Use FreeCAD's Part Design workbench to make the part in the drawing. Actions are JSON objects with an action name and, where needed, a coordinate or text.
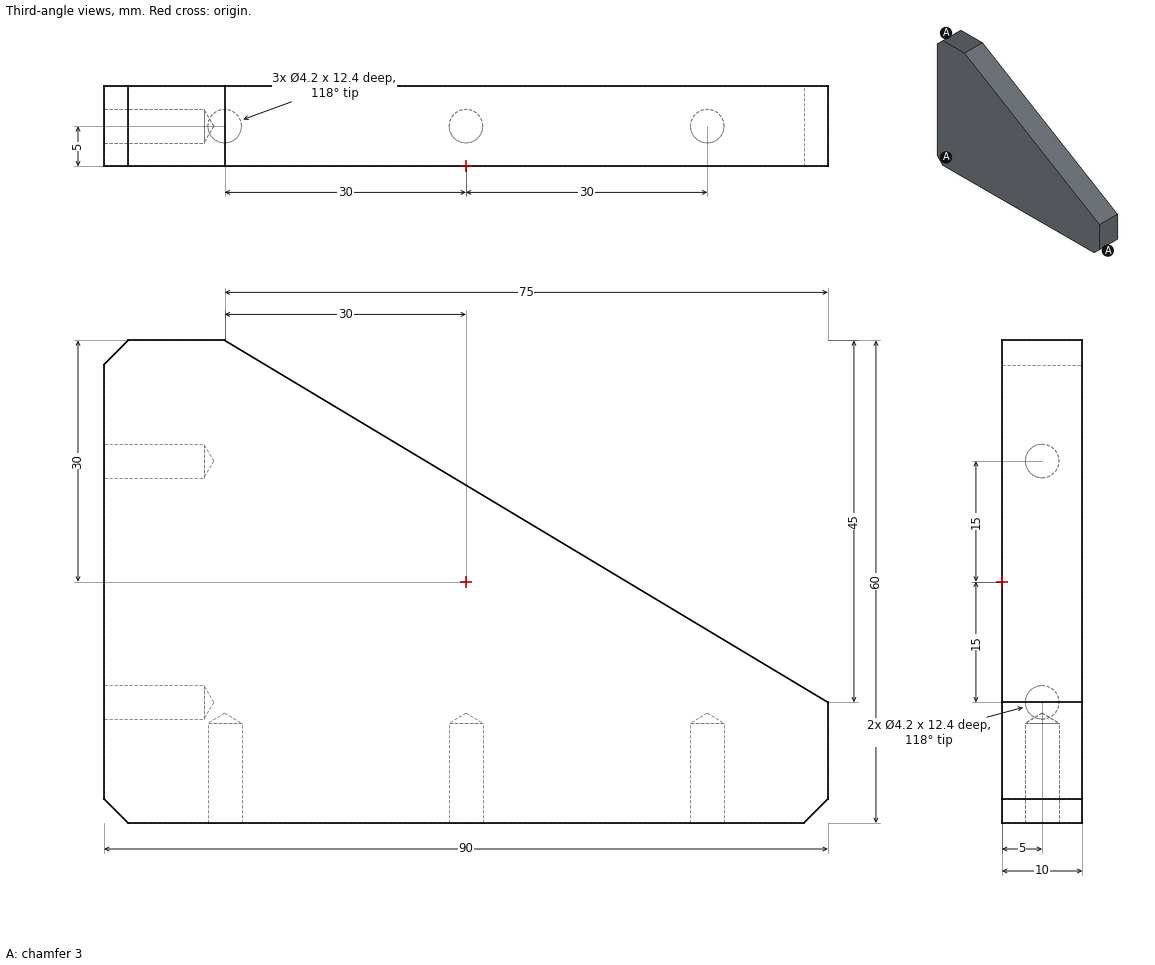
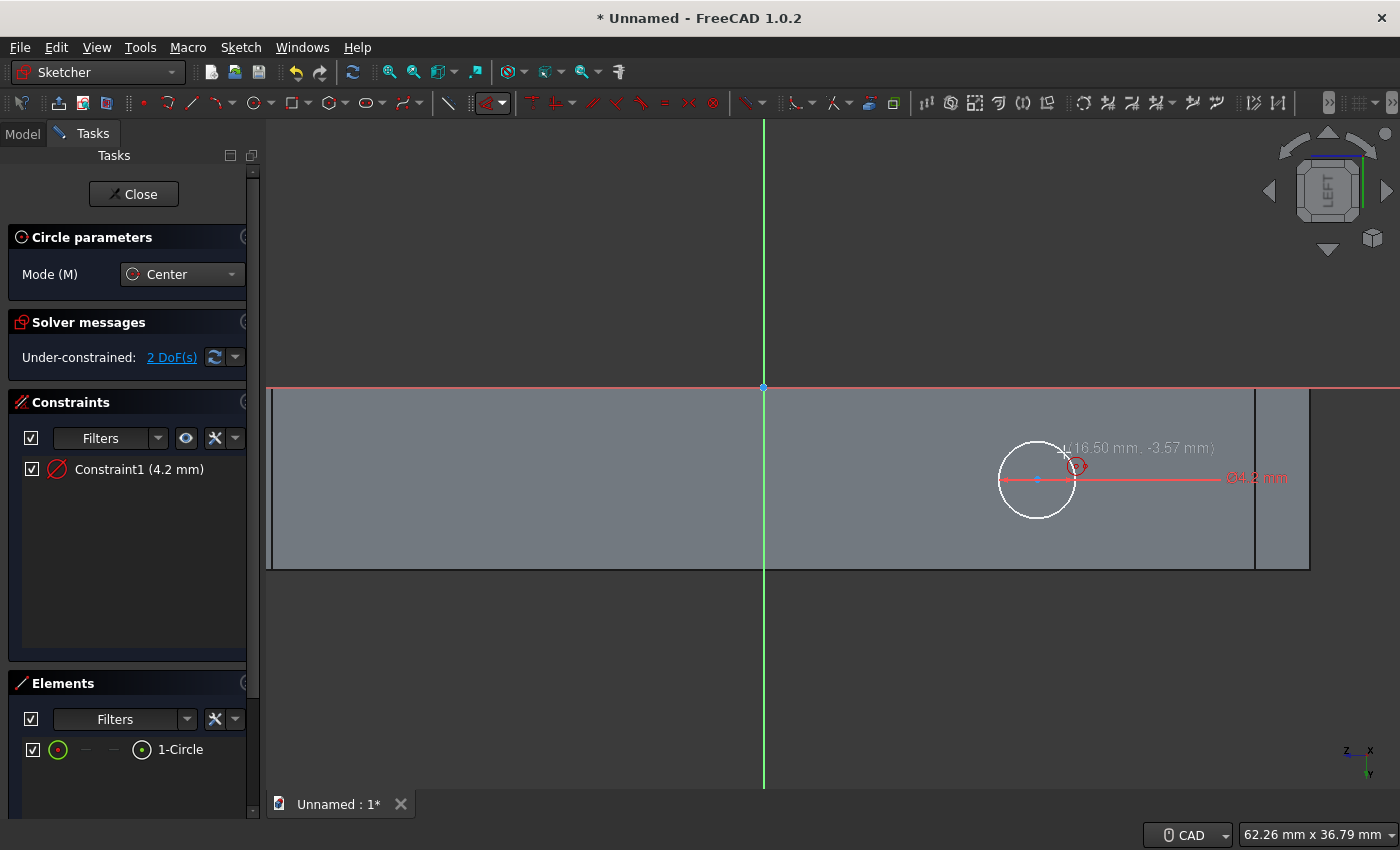
{"action": "left_click", "coordinate": [490, 479]}
{"action": "mouse_move", "coordinate": [517, 452]}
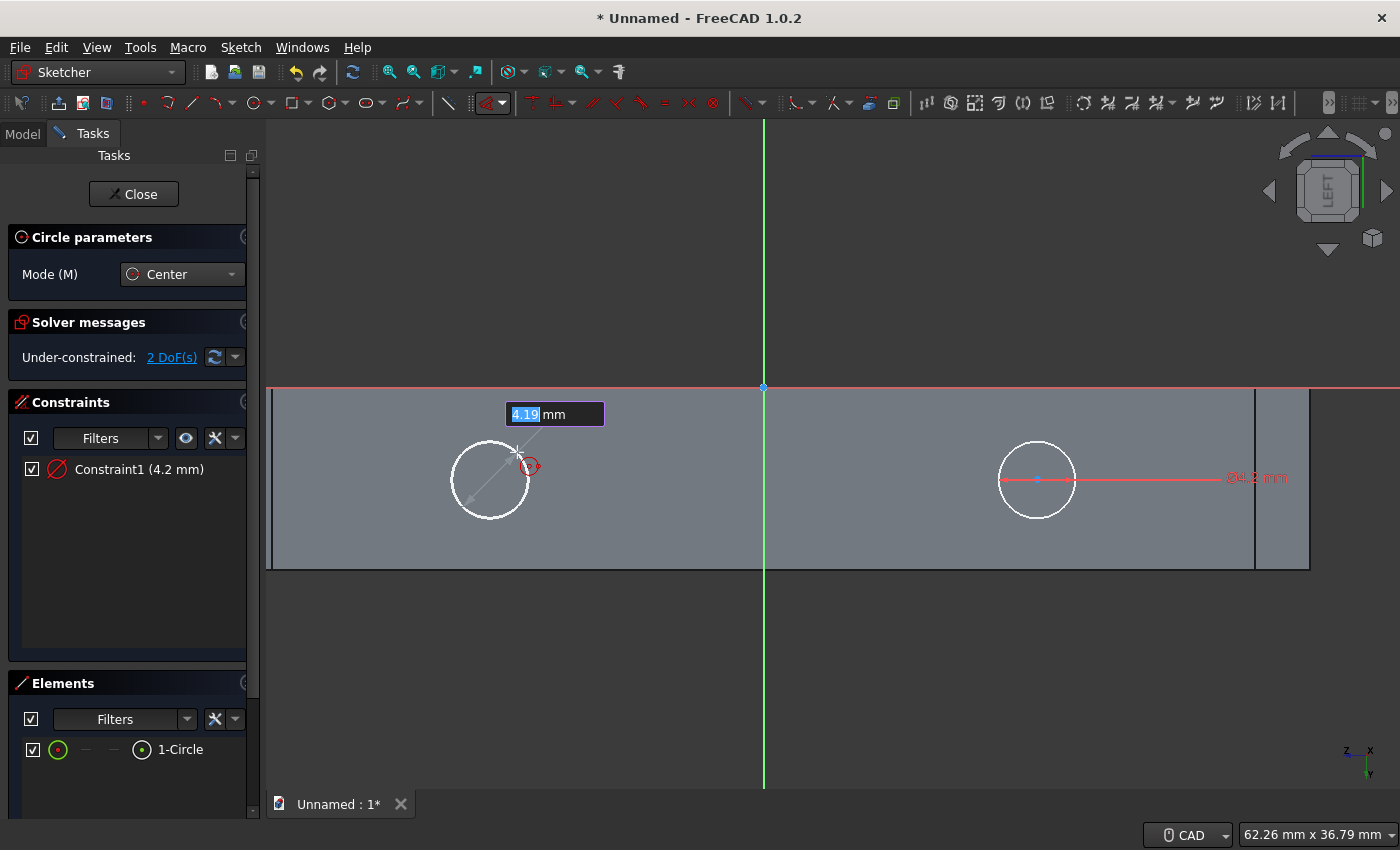
{"action": "type", "text": "4.2"}
{"action": "key", "text": "Return"}
{"action": "key", "text": "Escape"}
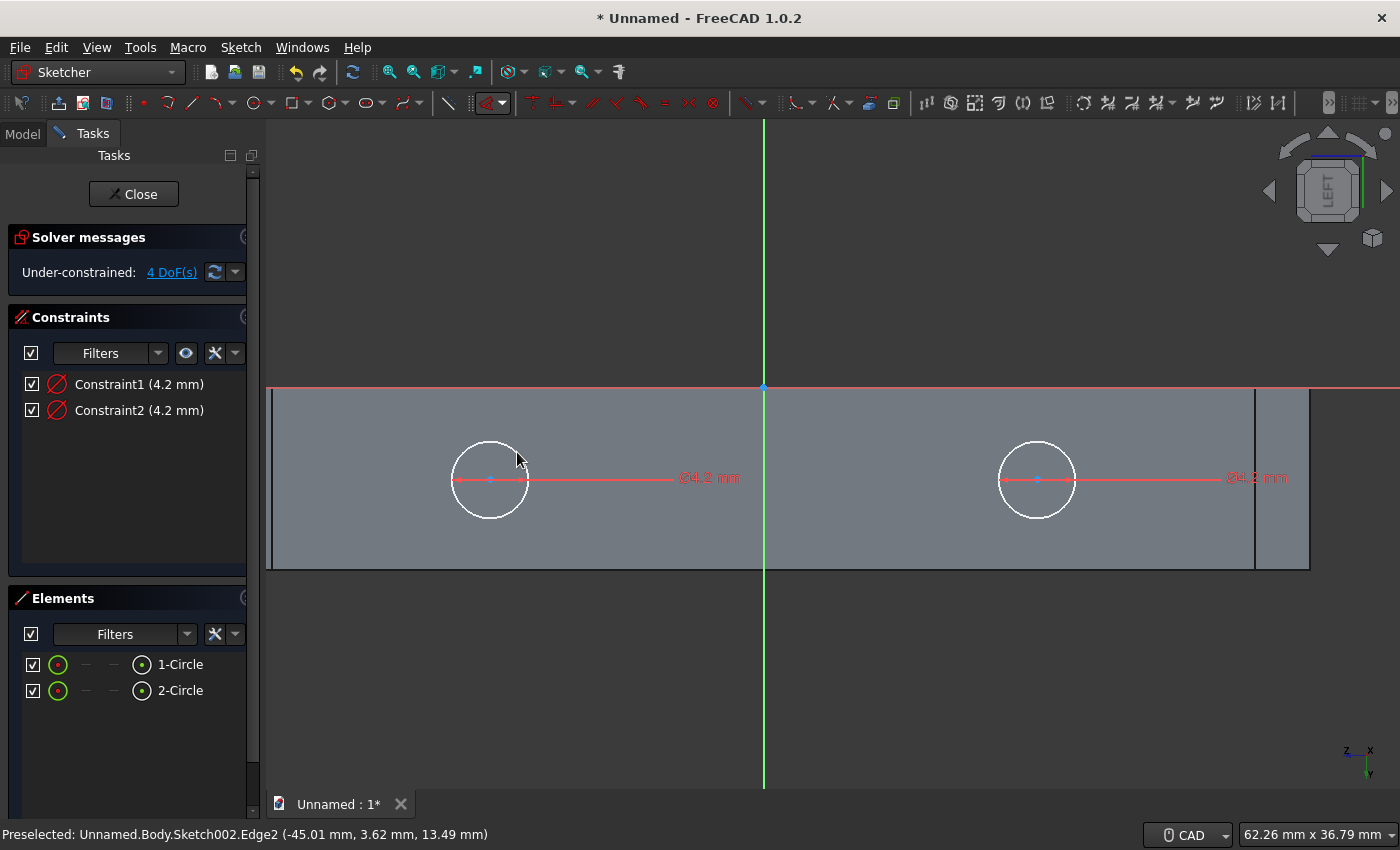
{"action": "left_click", "coordinate": [1037, 480]}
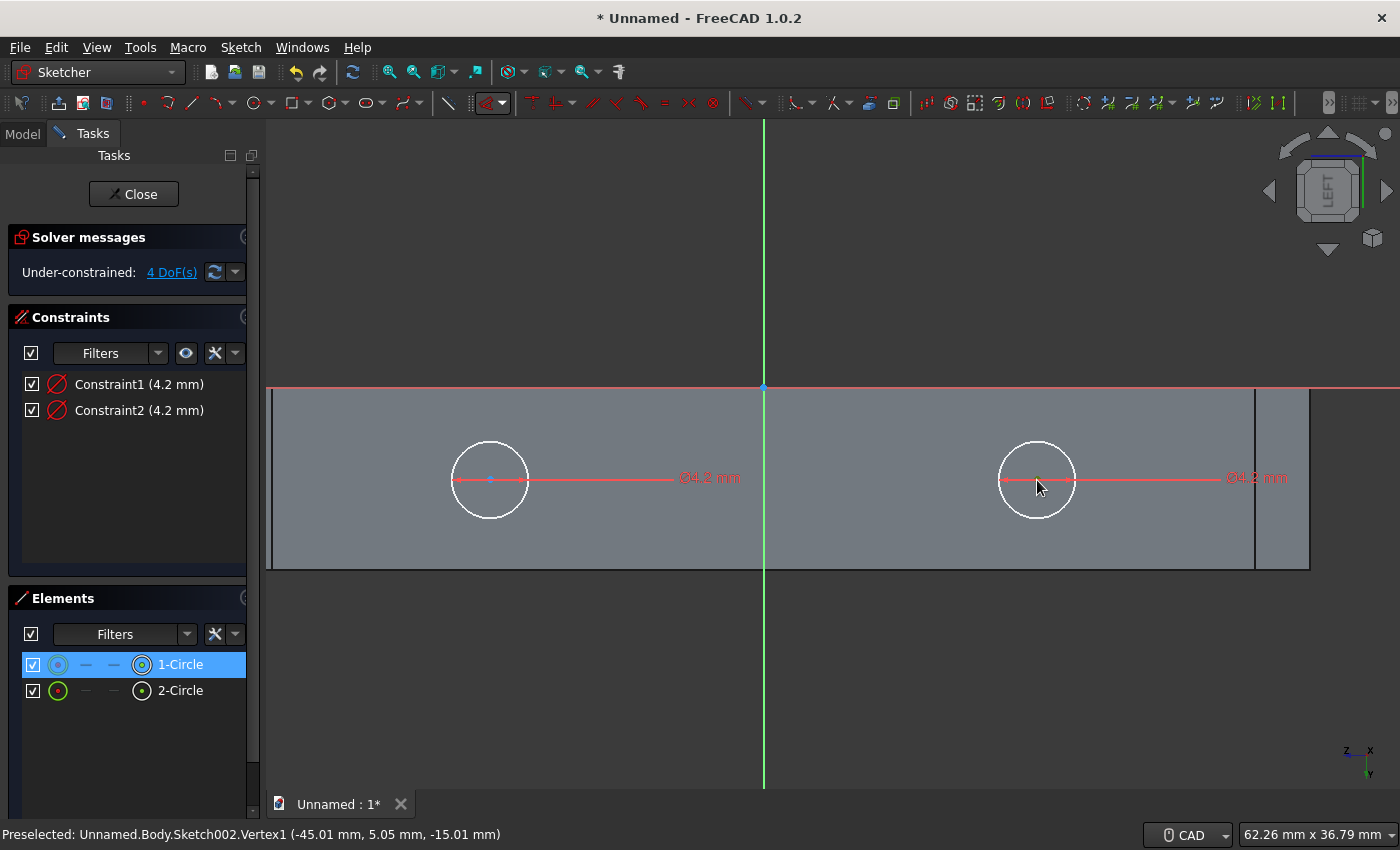
{"action": "left_click", "coordinate": [490, 480]}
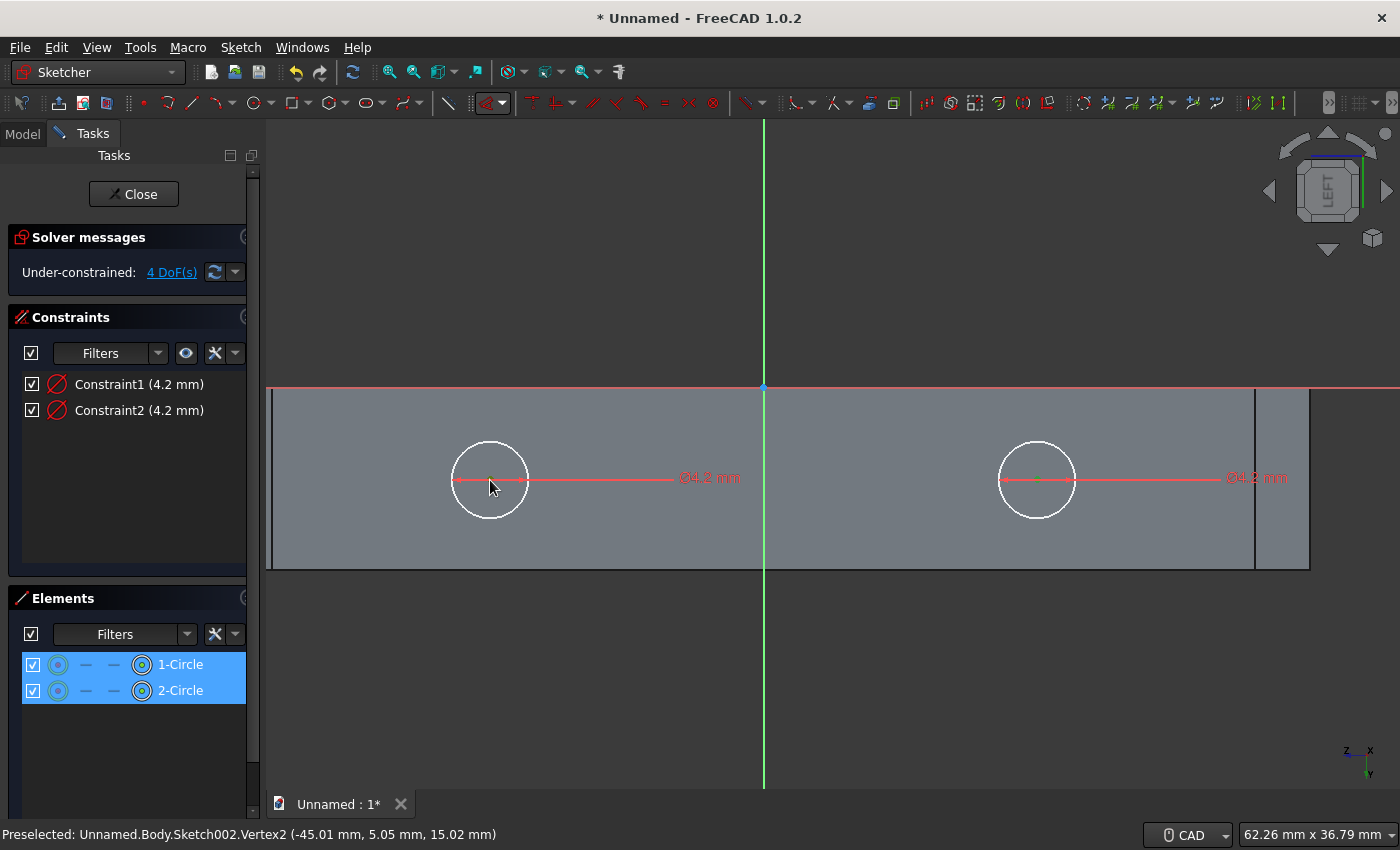
{"action": "key", "text": "h"}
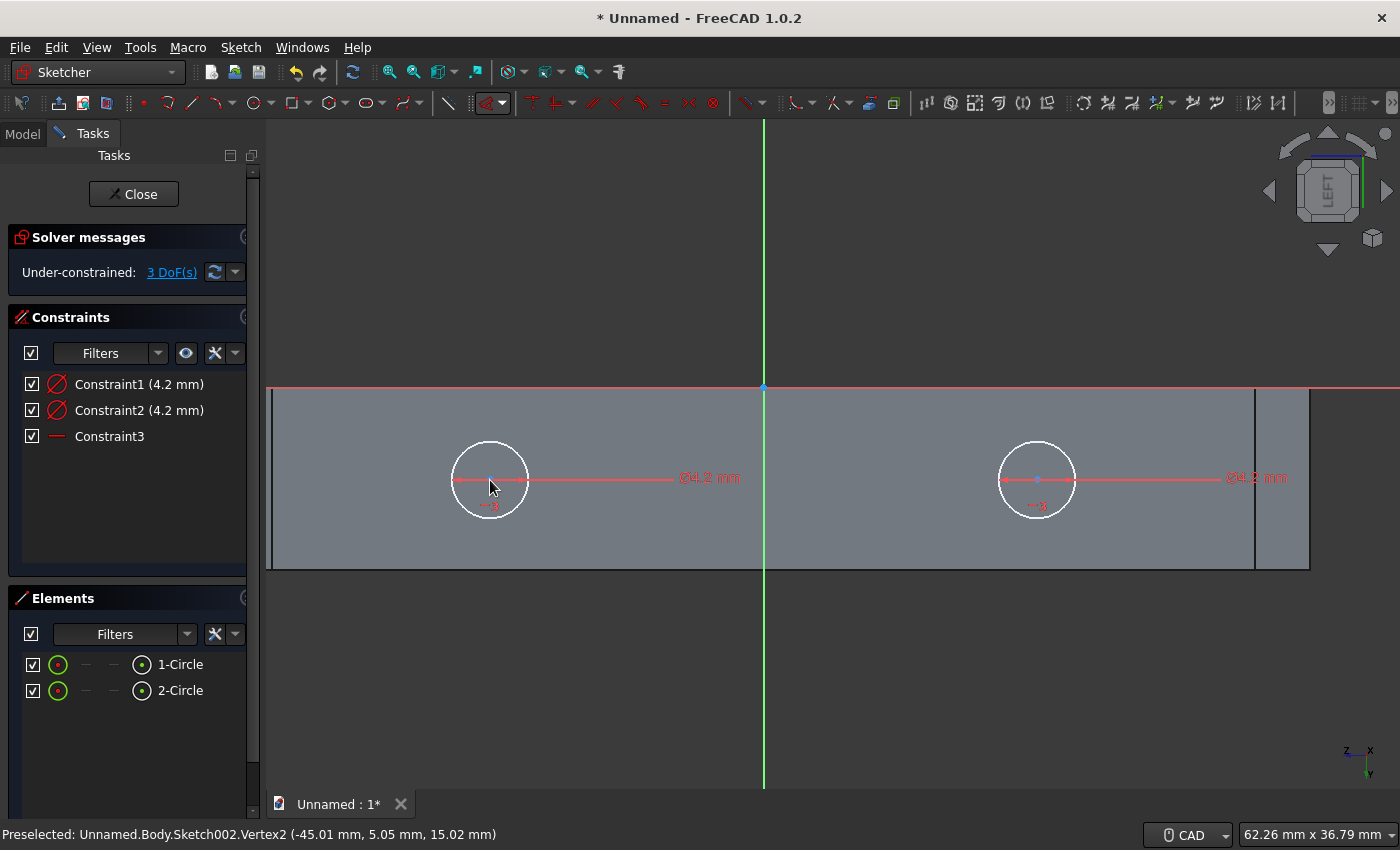
{"action": "key", "text": "d"}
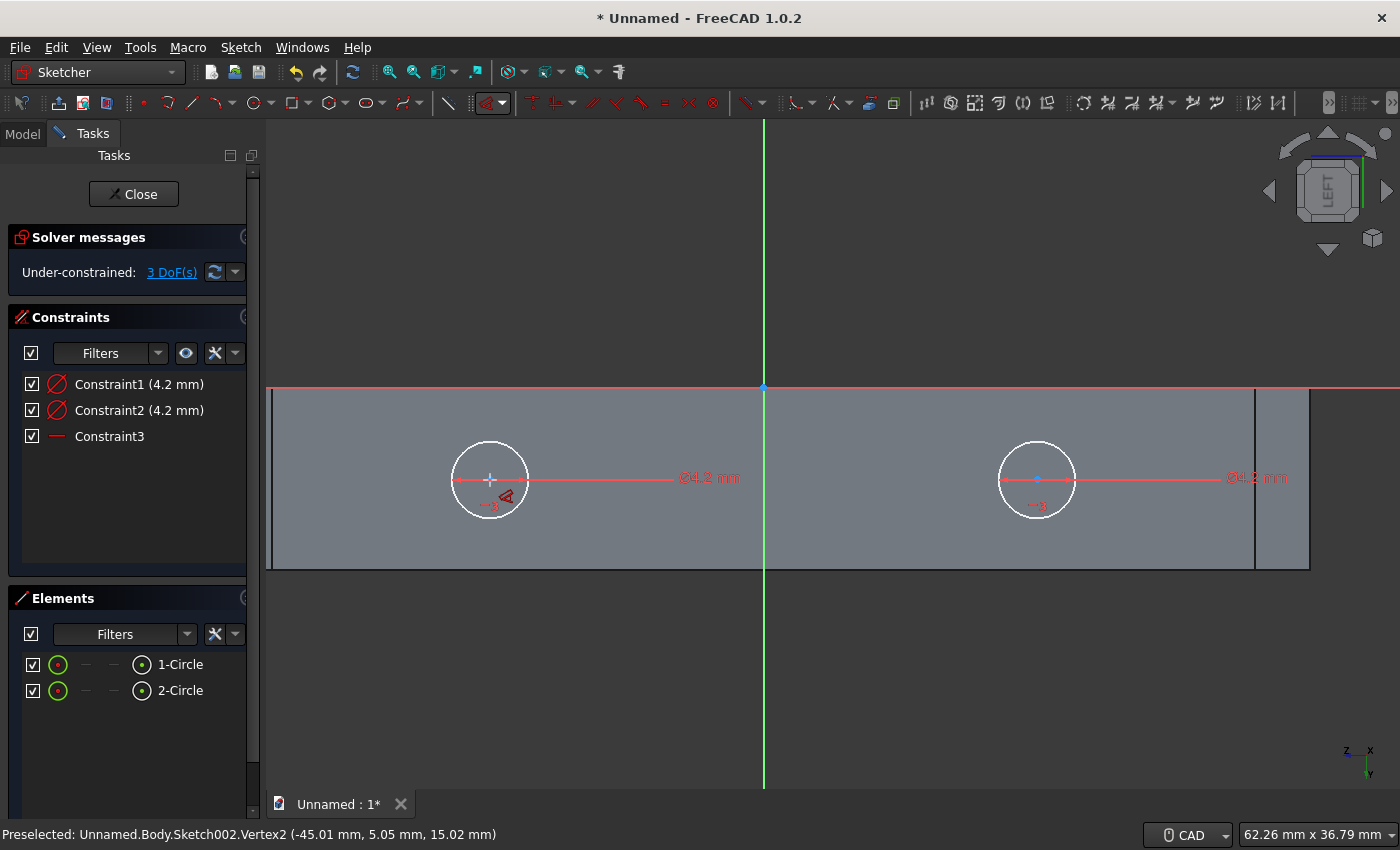
{"action": "left_click", "coordinate": [1037, 480]}
{"action": "left_click", "coordinate": [1071, 434]}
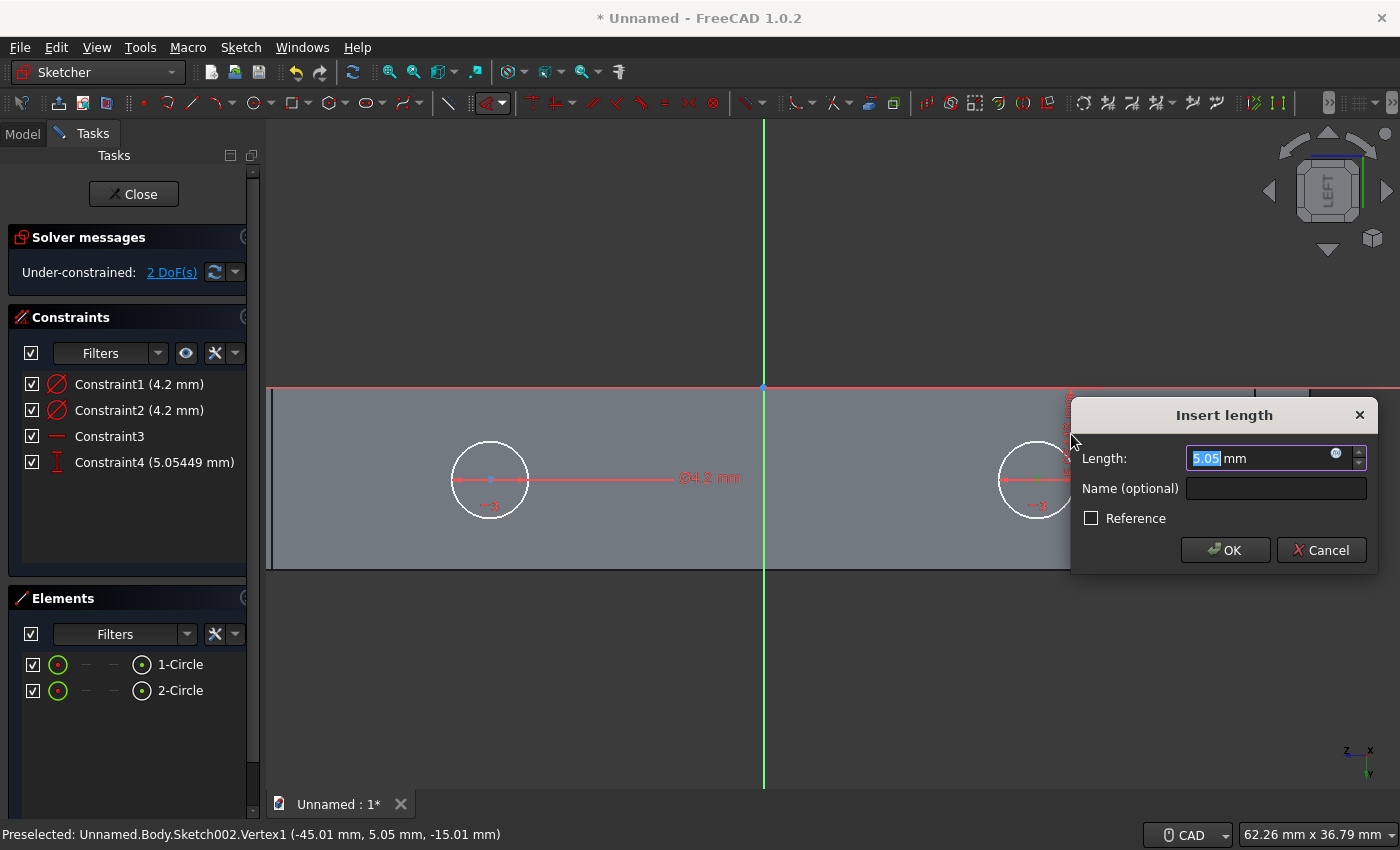
{"action": "type", "text": "5"}
{"action": "key", "text": "Return"}